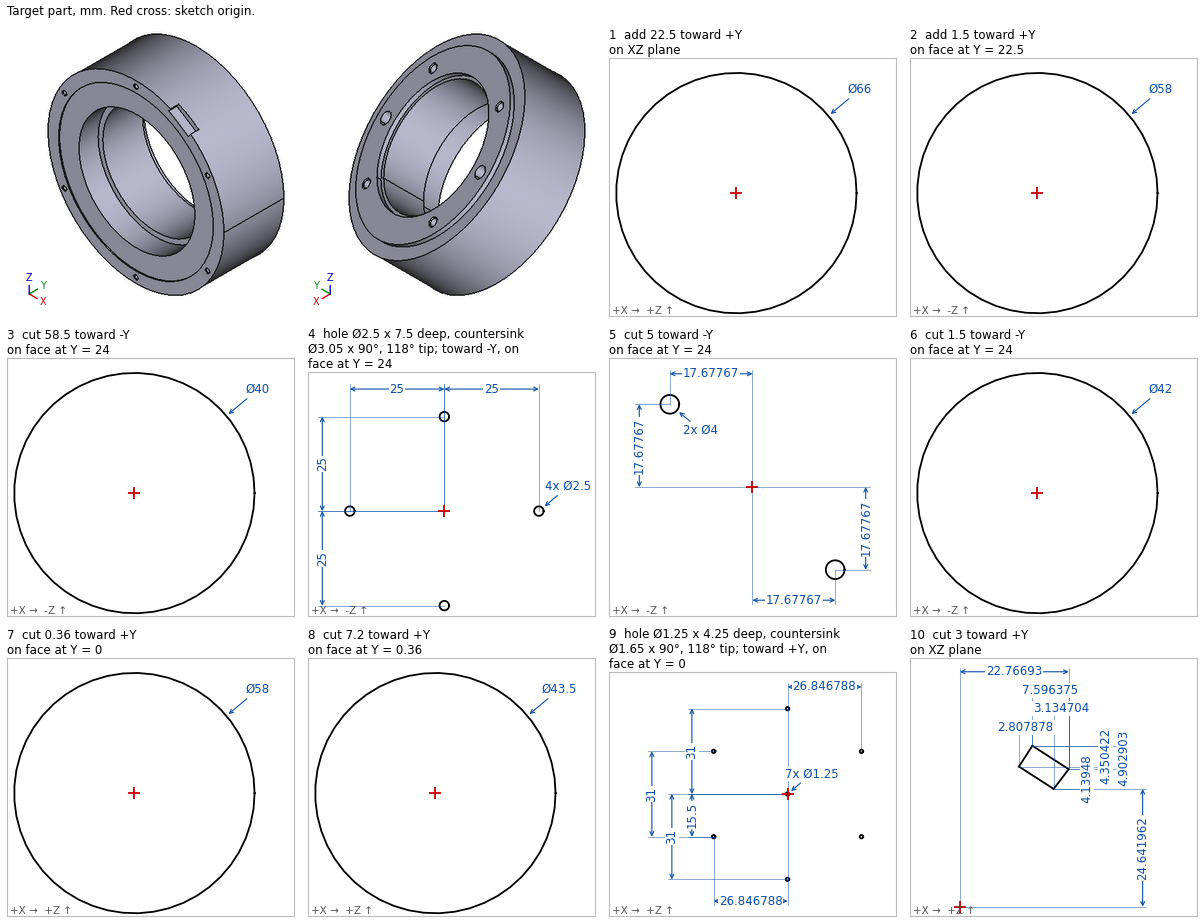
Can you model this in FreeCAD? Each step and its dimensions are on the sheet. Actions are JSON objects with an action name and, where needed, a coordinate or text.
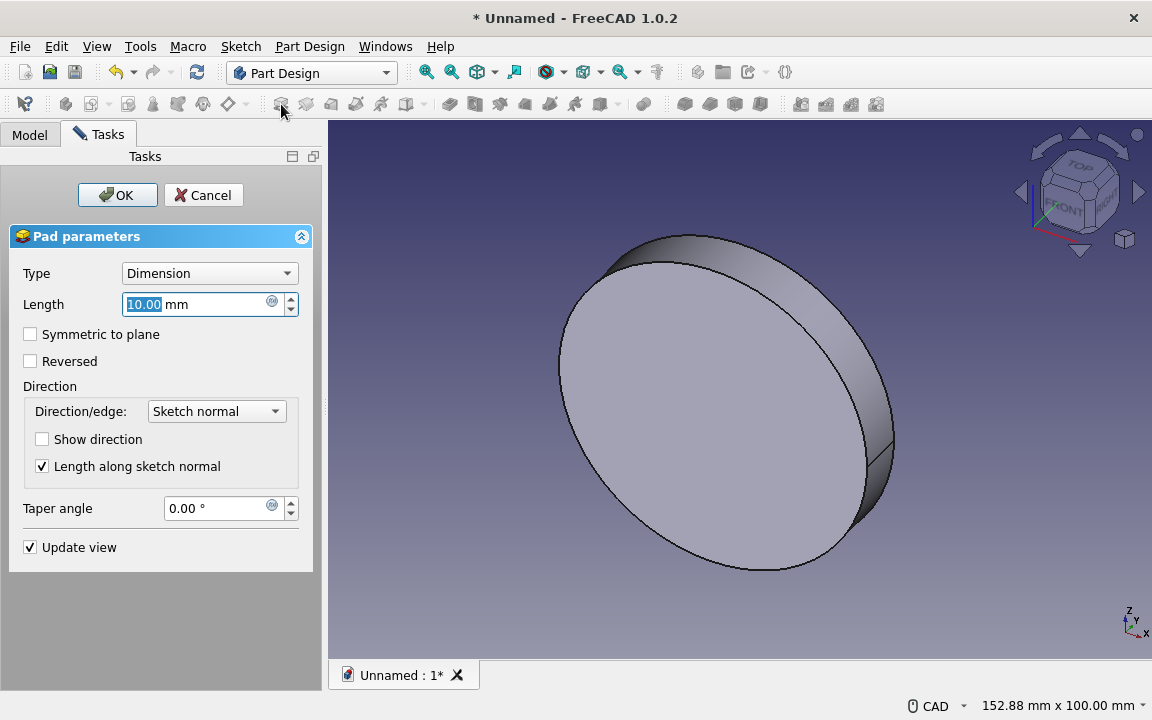
{"action": "type", "text": "22.5"}
{"action": "key", "text": "Tab"}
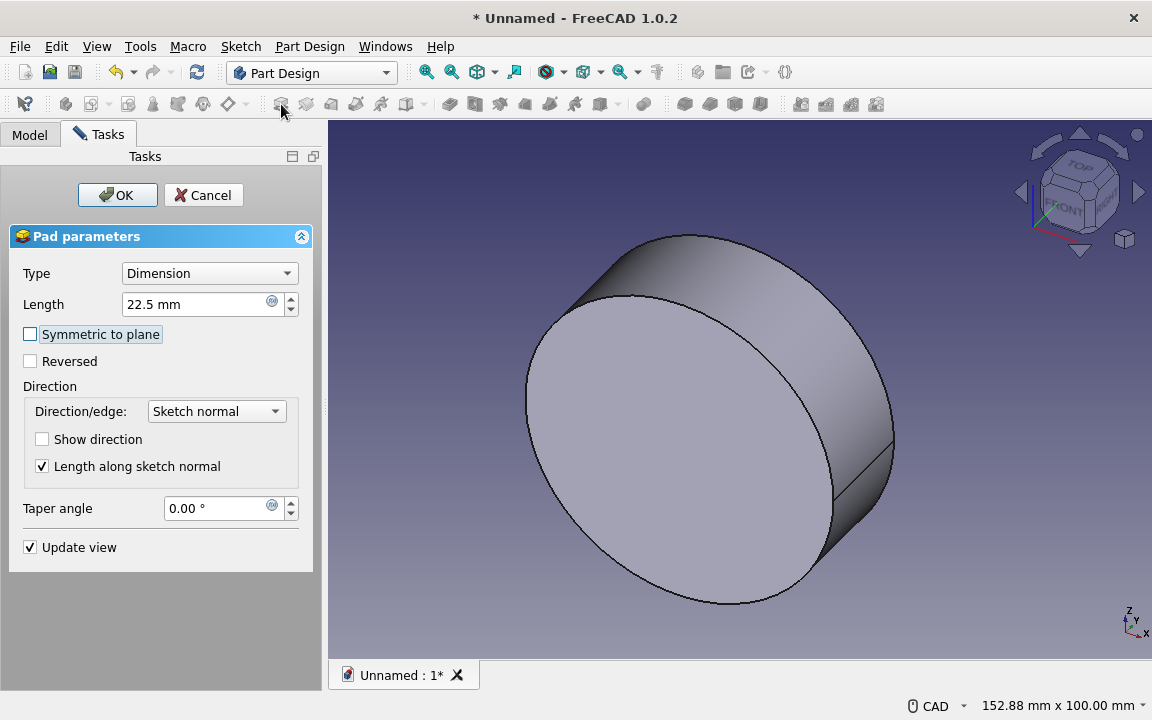
{"action": "left_click", "coordinate": [31, 361]}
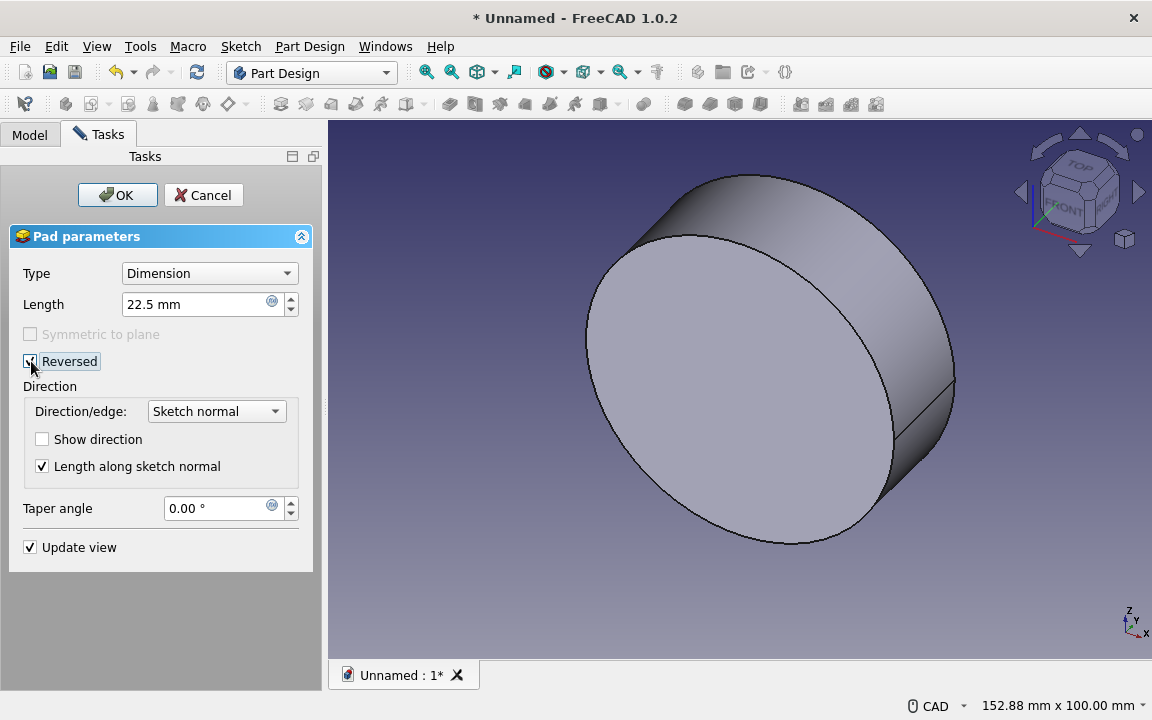
{"action": "left_click", "coordinate": [118, 195]}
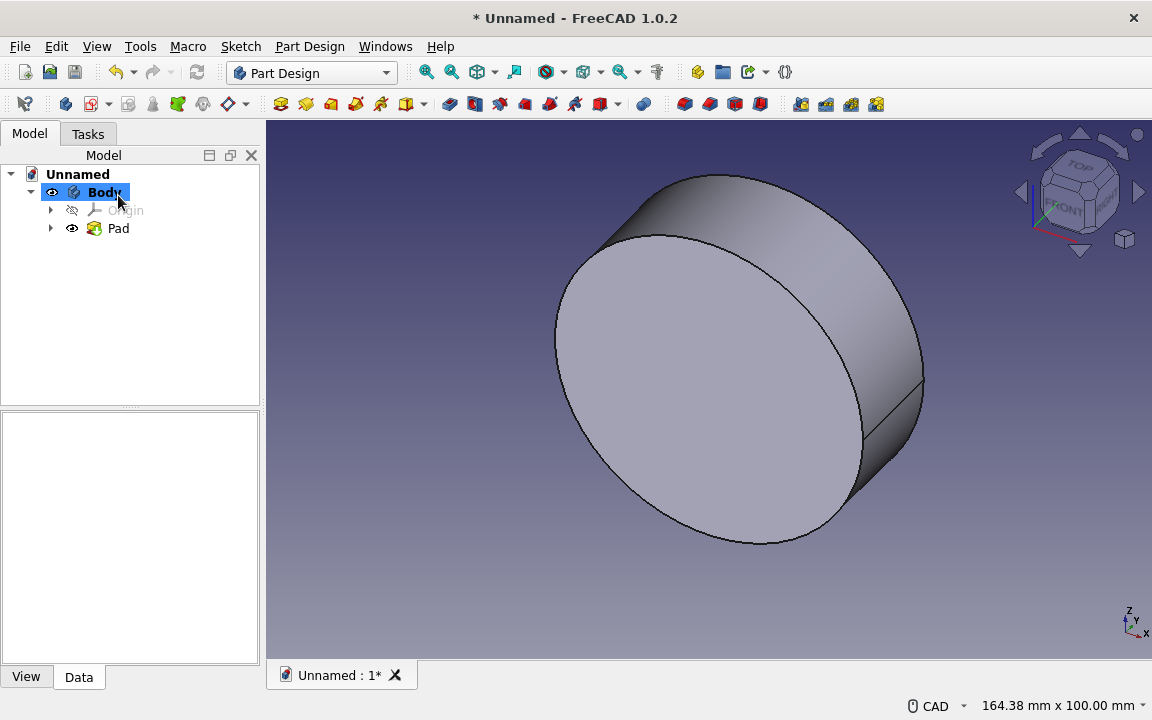
{"action": "key", "text": "4"}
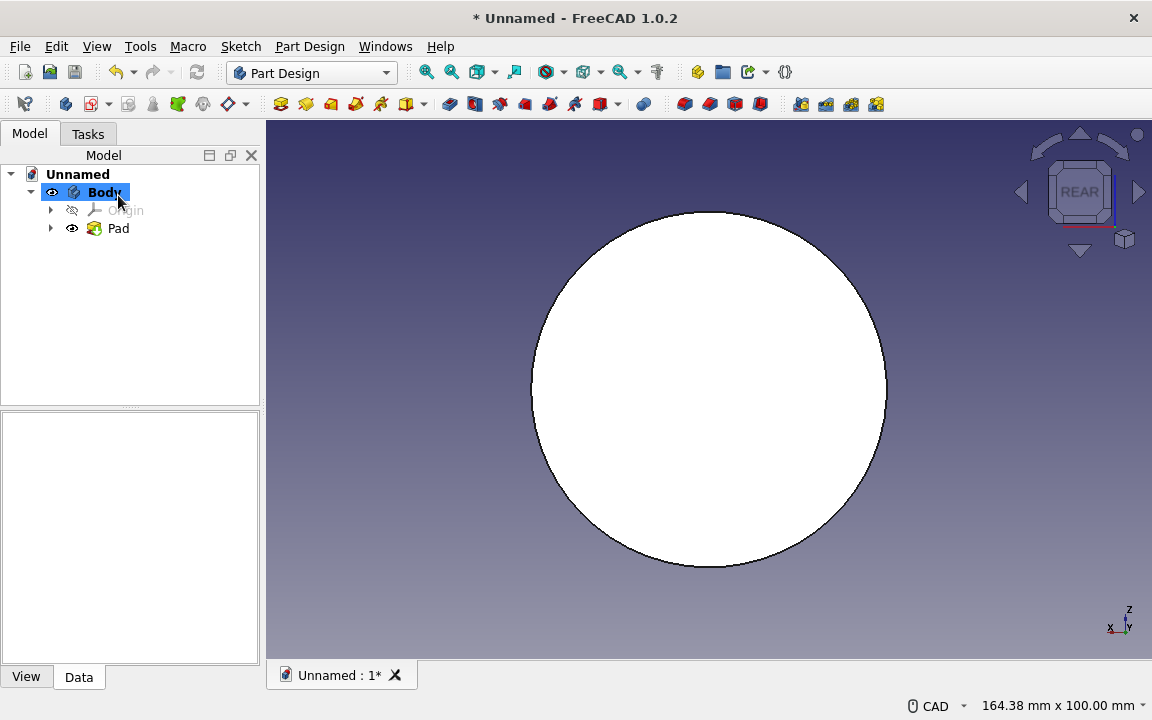
{"action": "left_click", "coordinate": [709, 388]}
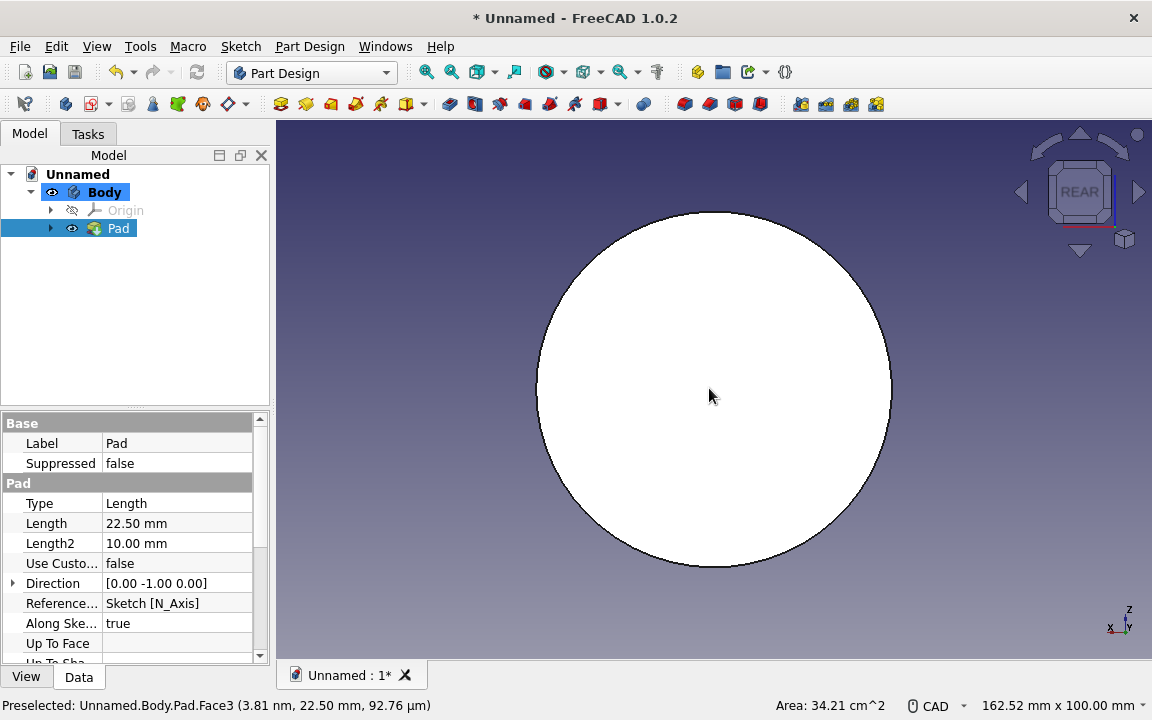
{"action": "left_click", "coordinate": [90, 104]}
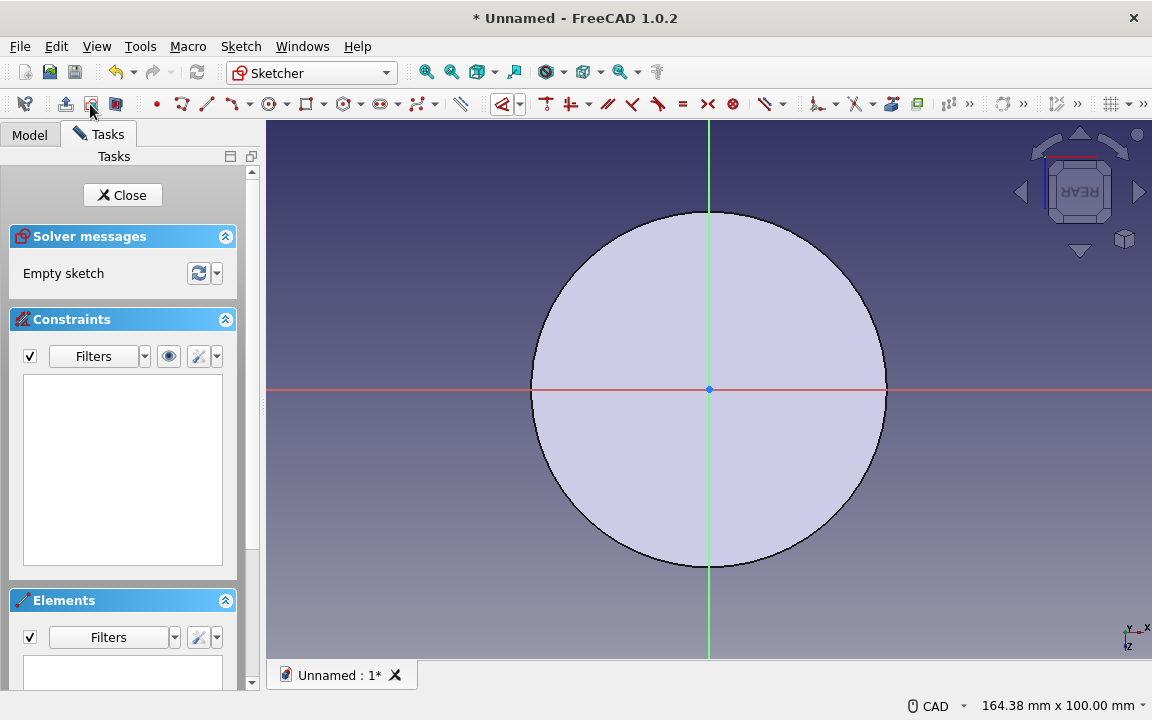
{"action": "left_click", "coordinate": [268, 104]}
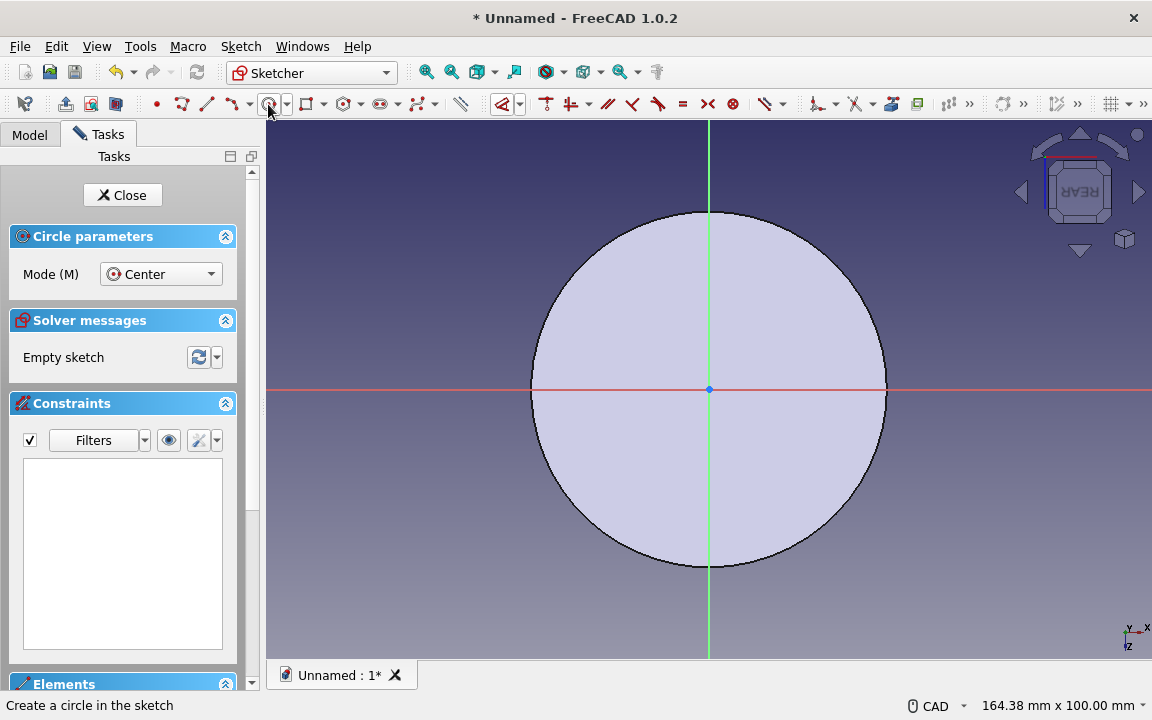
{"action": "left_click", "coordinate": [709, 390]}
{"action": "left_click", "coordinate": [820, 279]}
{"action": "key", "text": "Escape"}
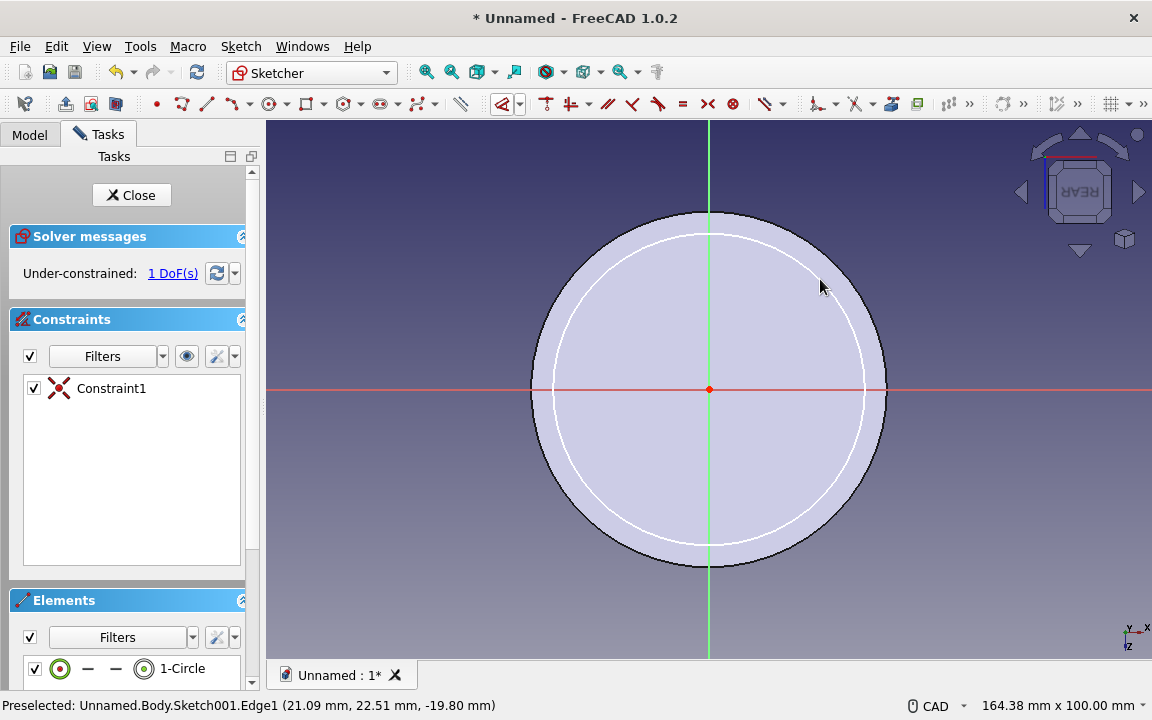
{"action": "left_click", "coordinate": [819, 279]}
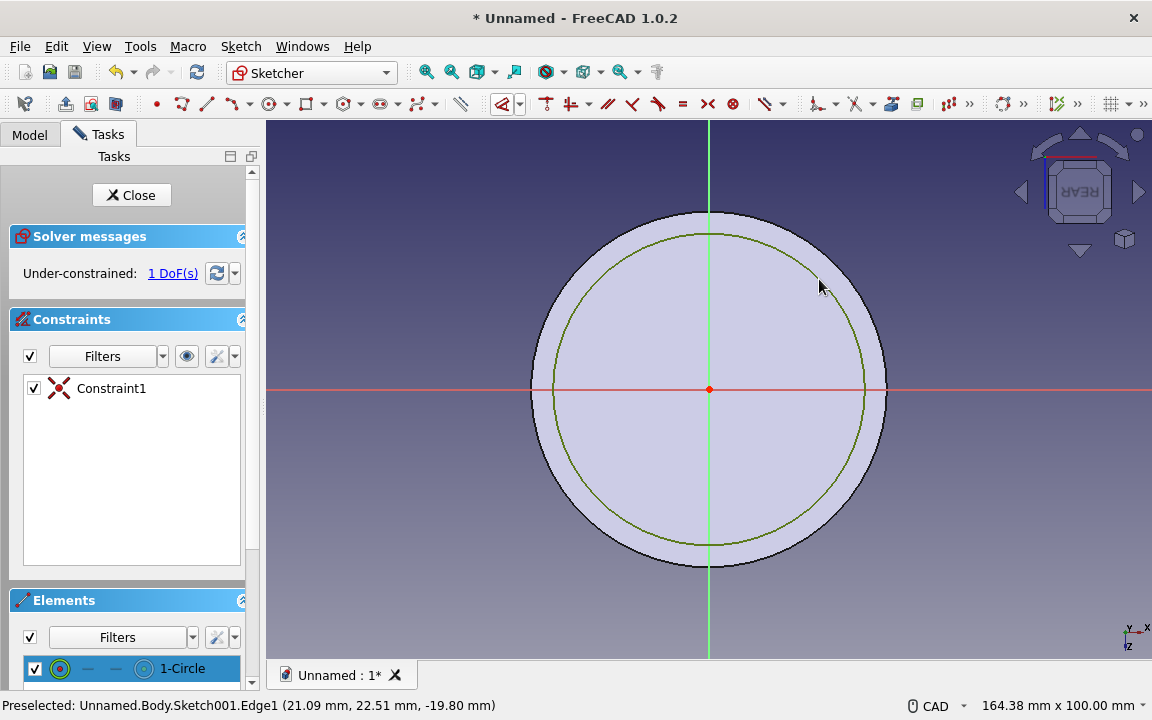
{"action": "left_click", "coordinate": [520, 104]}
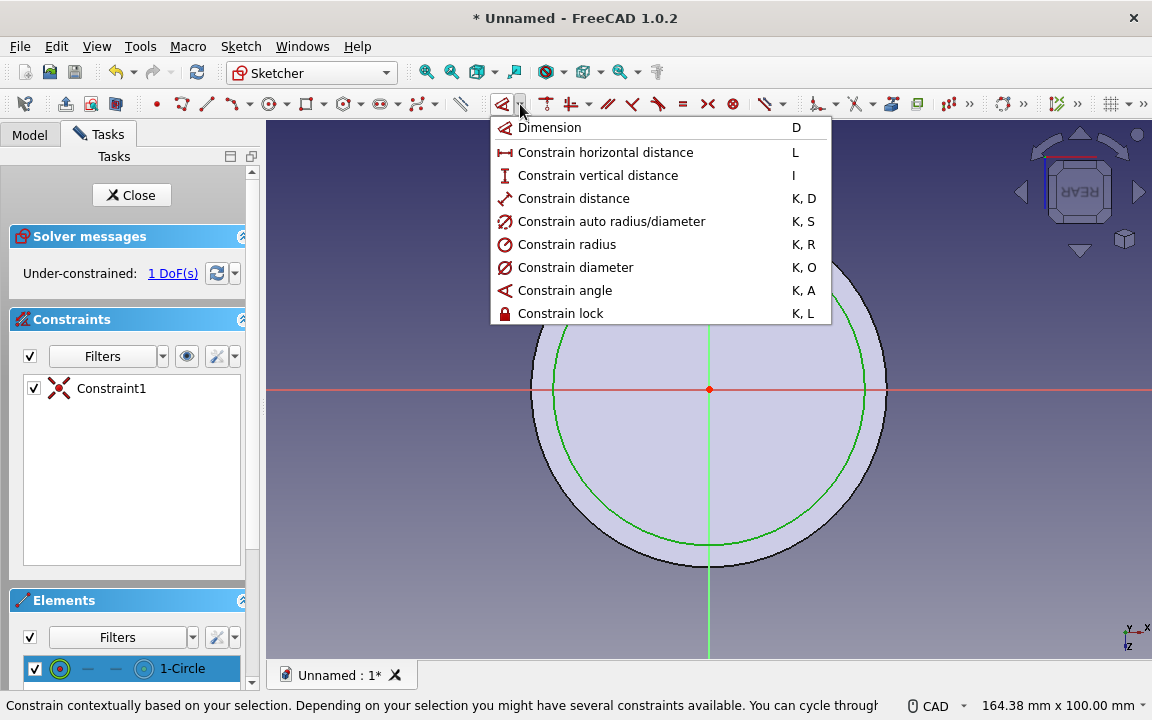
{"action": "left_click", "coordinate": [661, 268]}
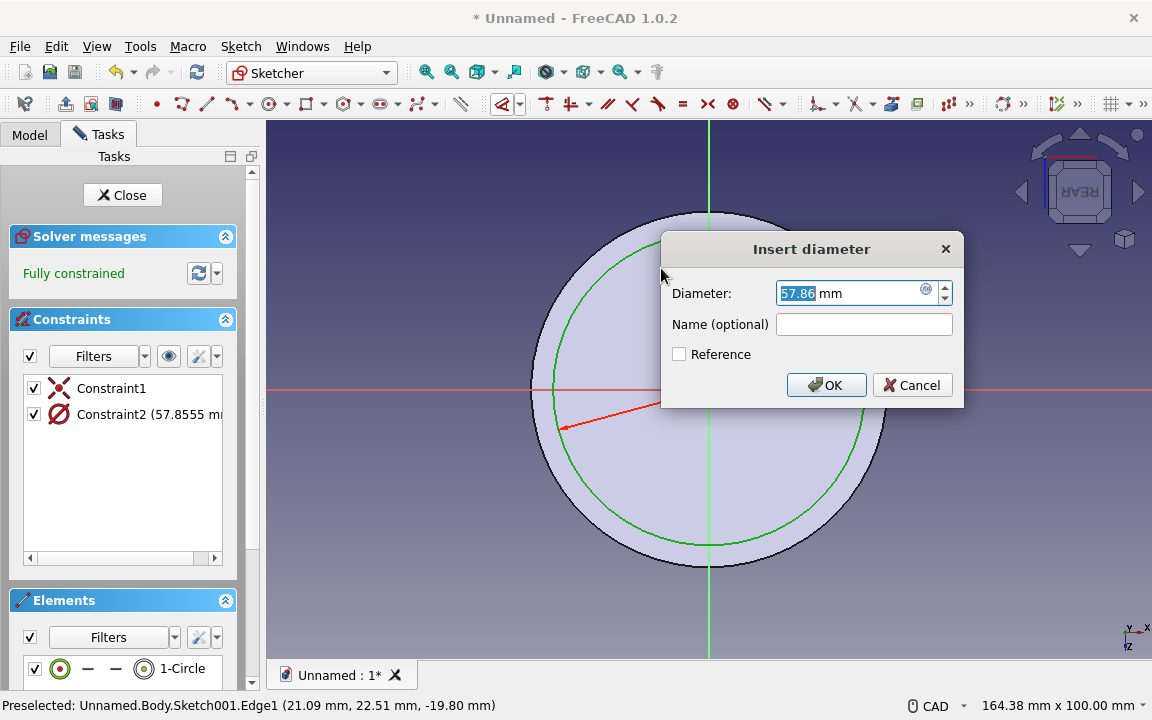
{"action": "type", "text": "58"}
{"action": "key", "text": "Return"}